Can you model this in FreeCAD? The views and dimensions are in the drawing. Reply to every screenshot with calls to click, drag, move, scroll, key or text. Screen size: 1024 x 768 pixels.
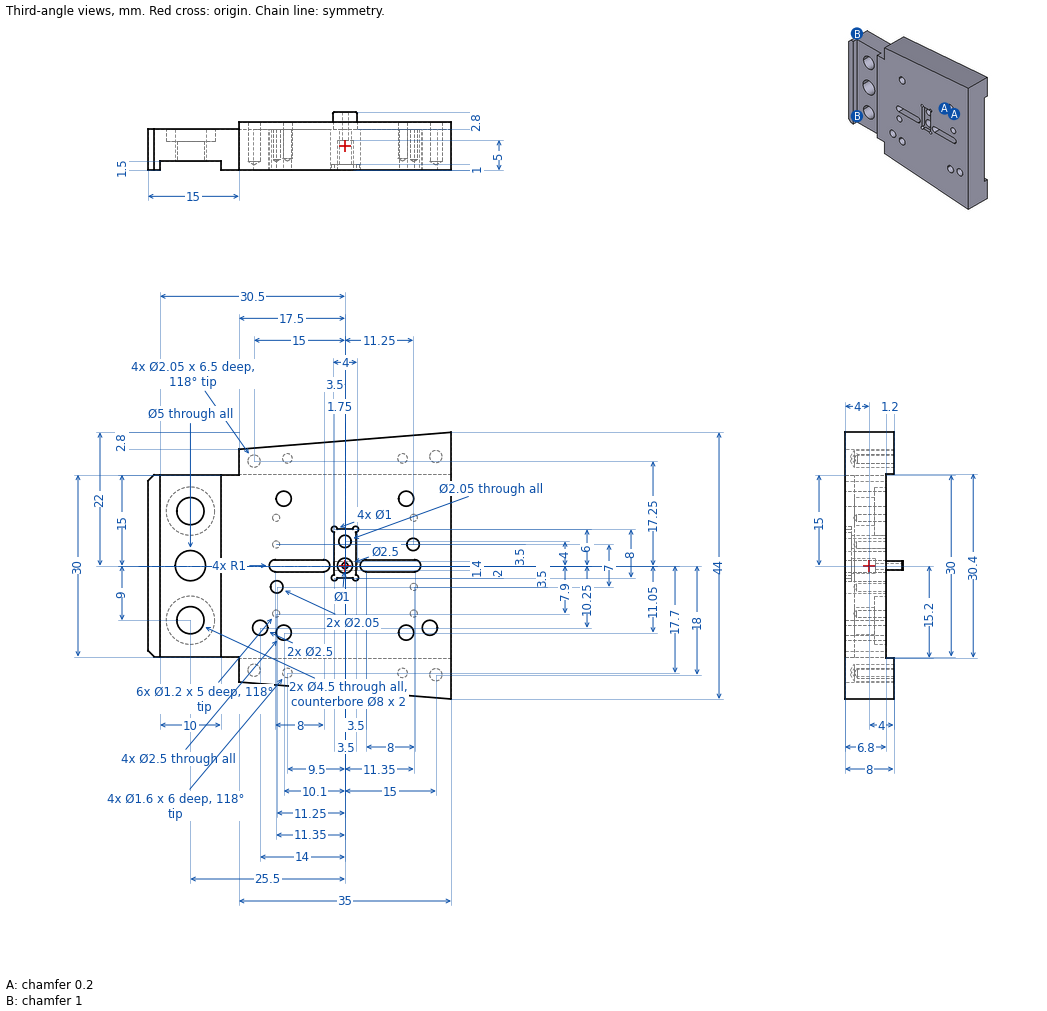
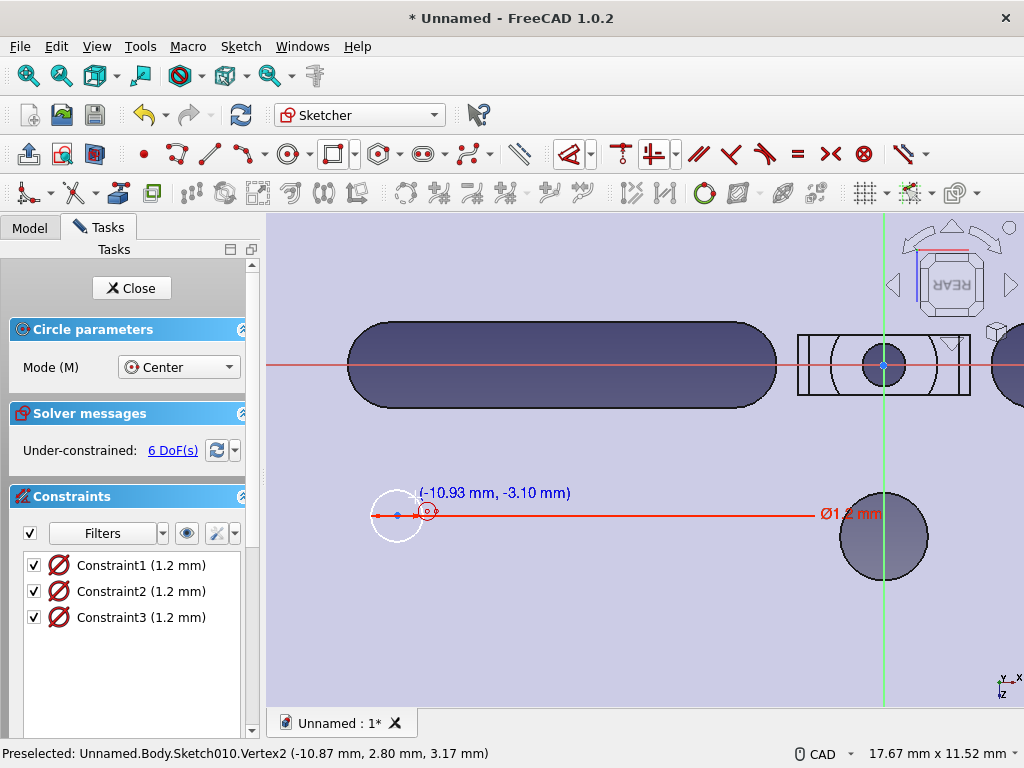
scroll(398, 515, down, 5)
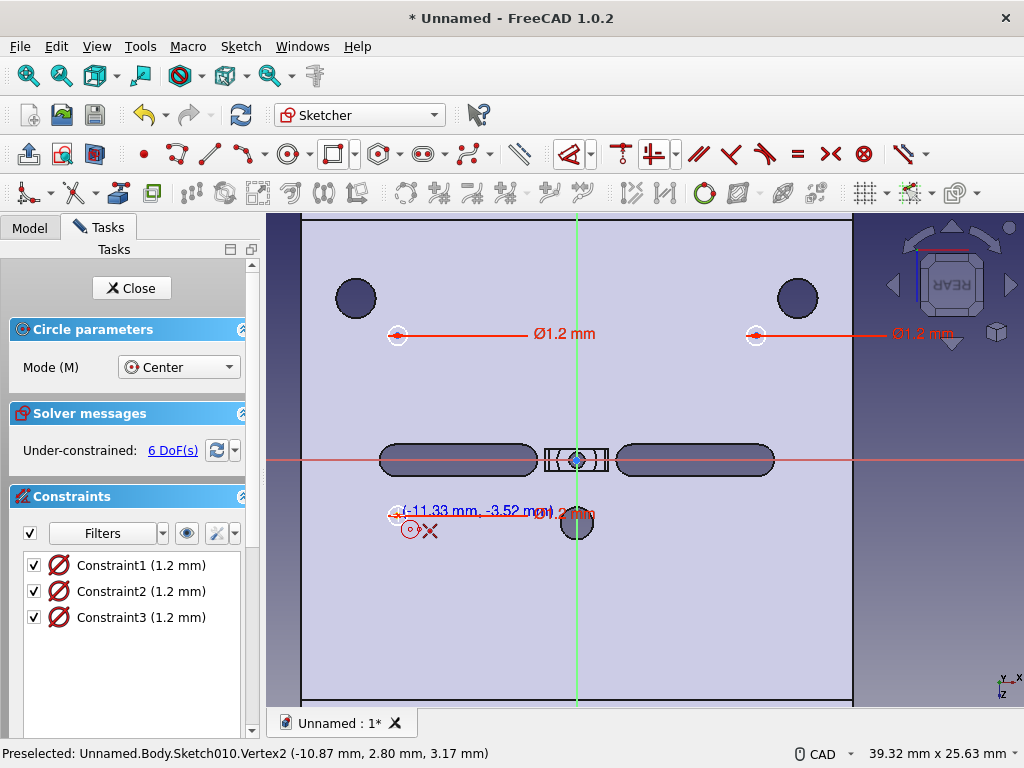
scroll(756, 405, up, 5)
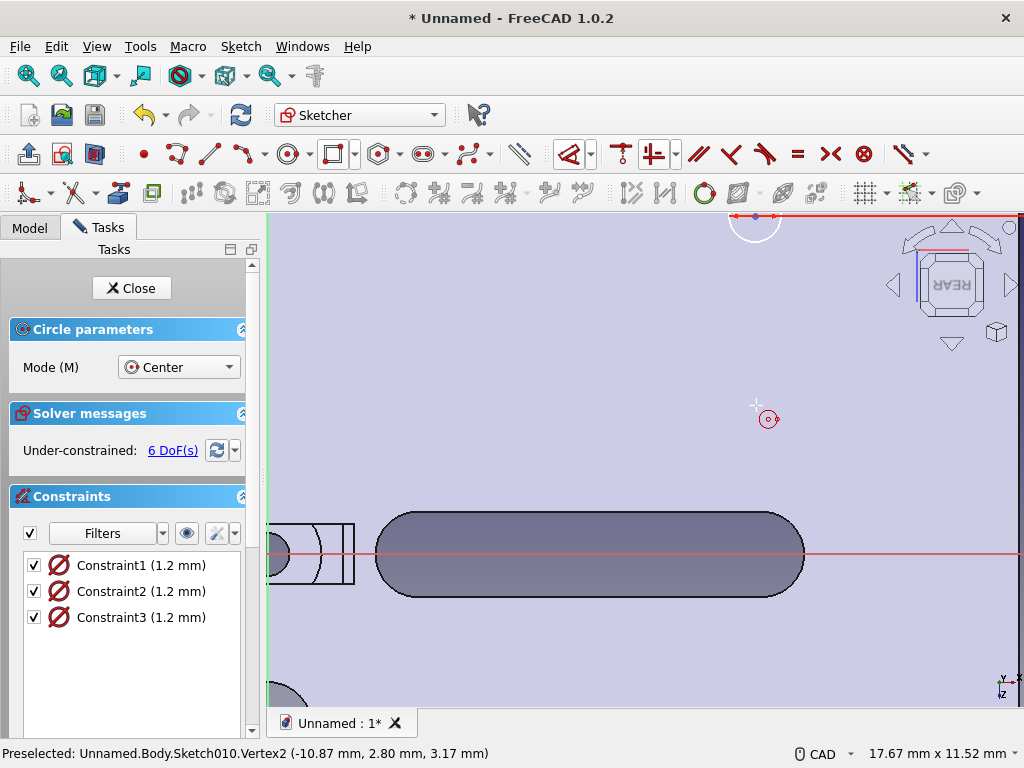
click(755, 404)
move(773, 386)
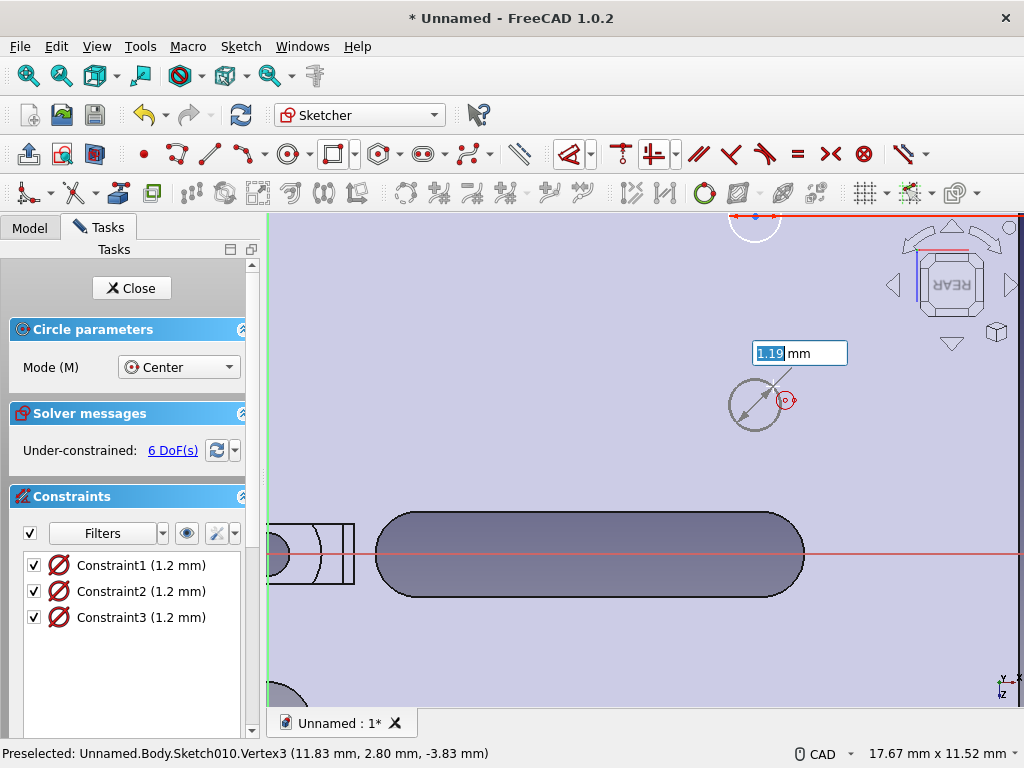
text(1.2)
key(Return)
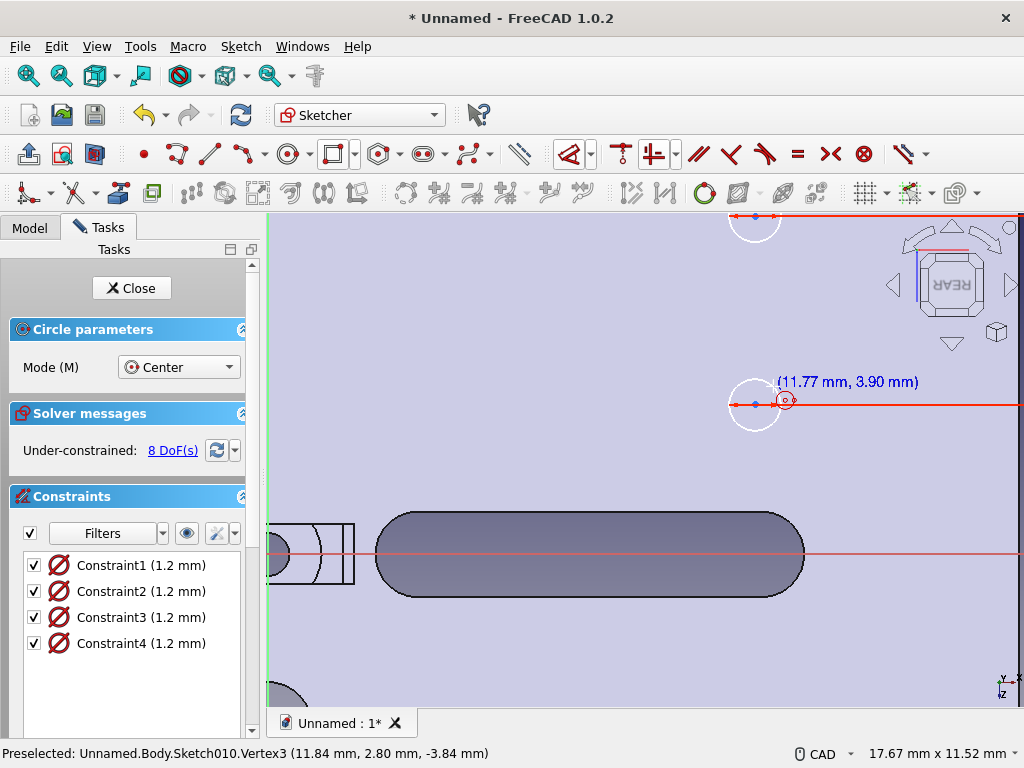
scroll(756, 405, down, 5)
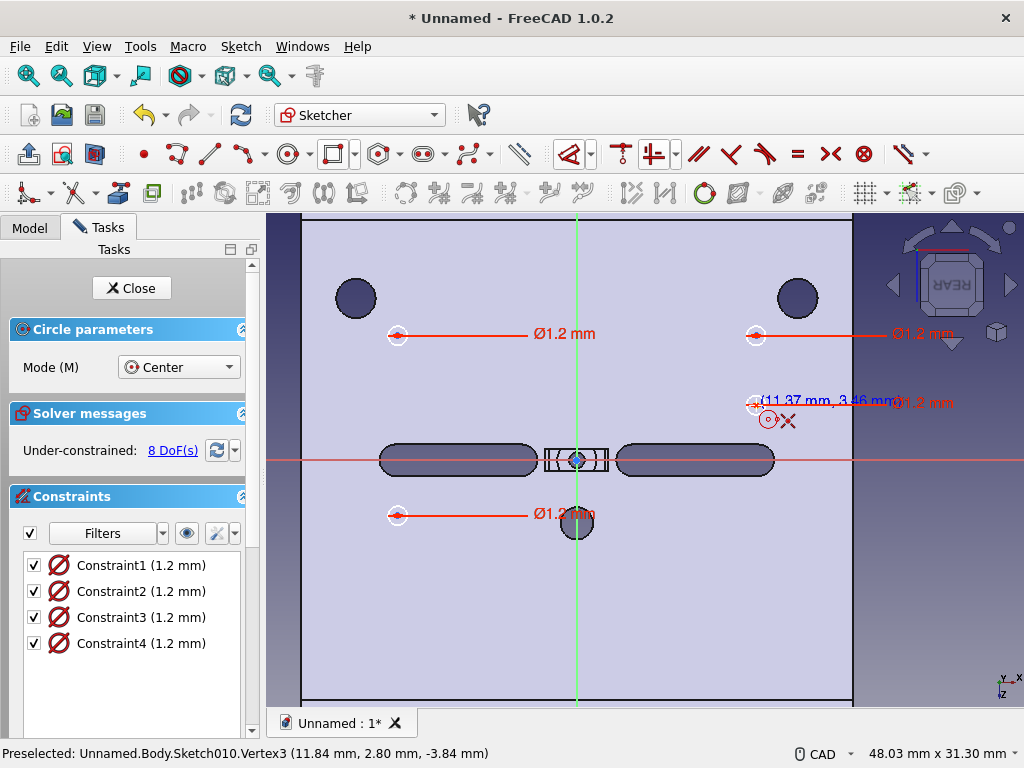
scroll(756, 585, up, 5)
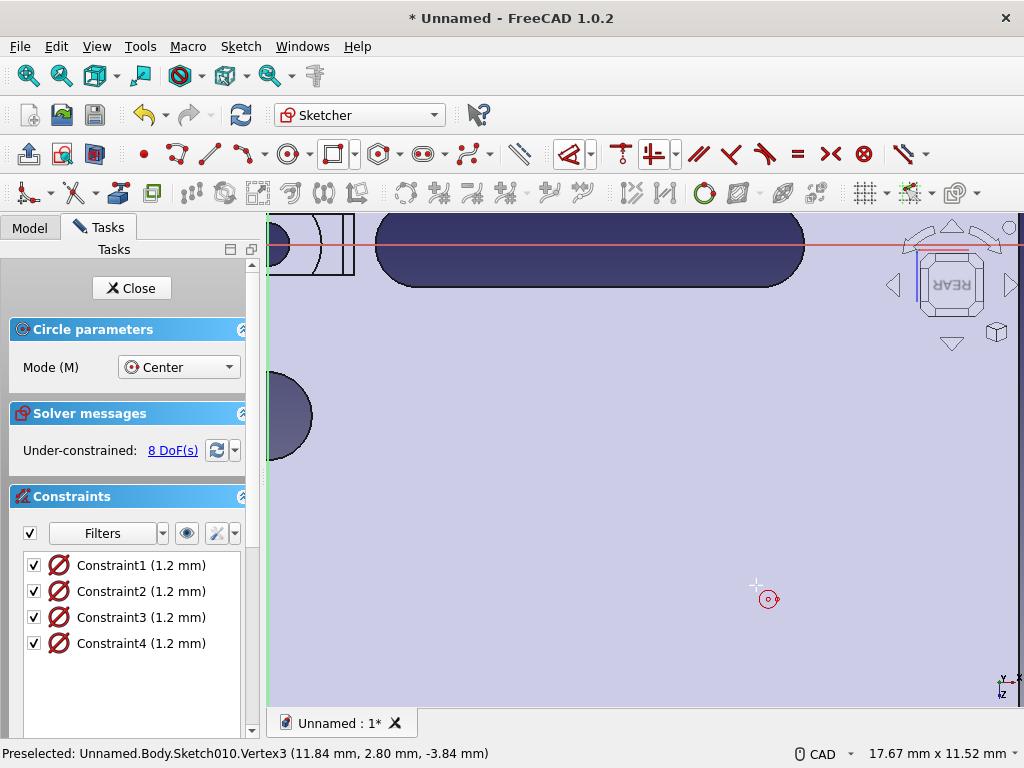
click(755, 583)
move(773, 565)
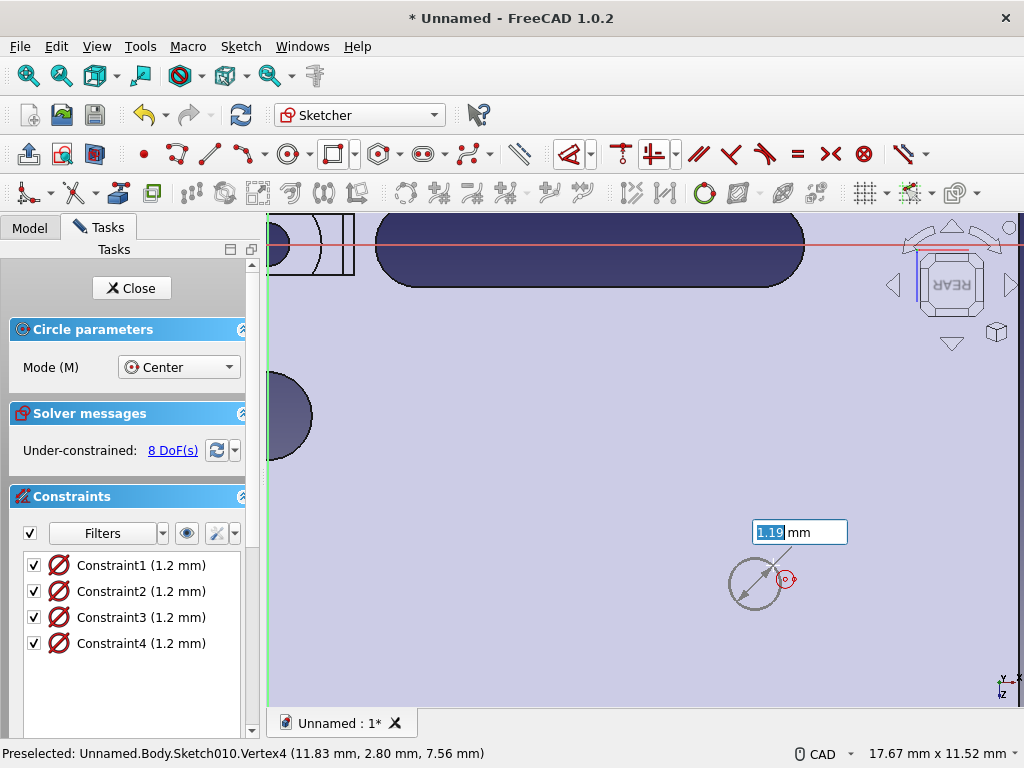
text(1.2)
key(Return)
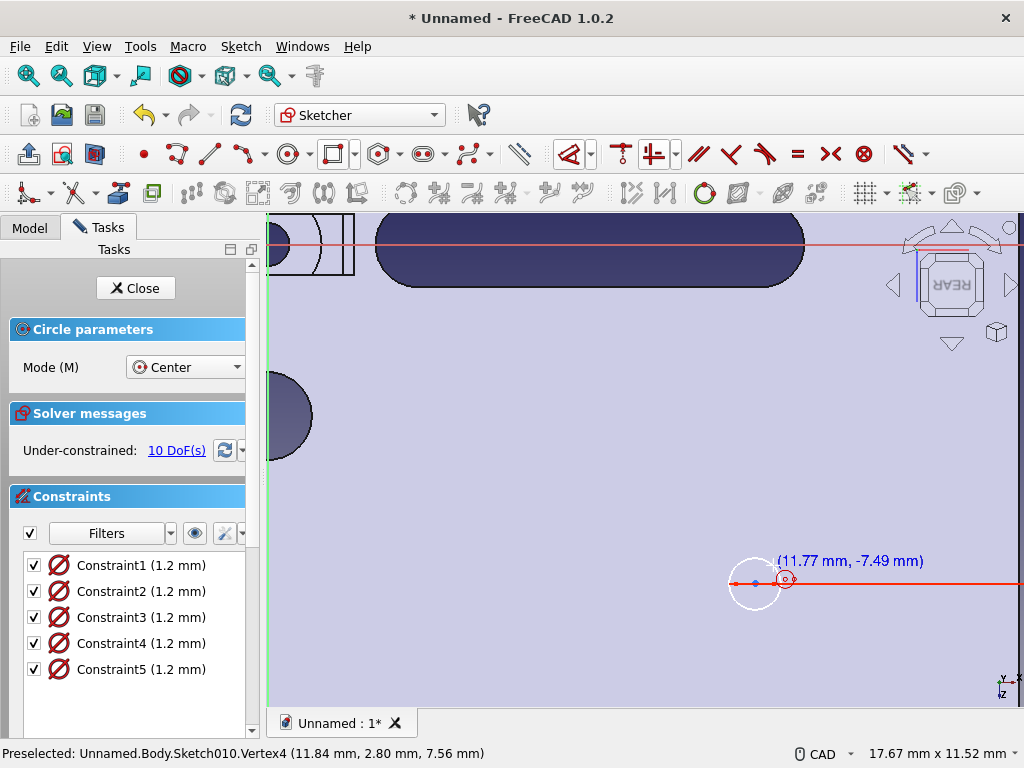
scroll(756, 585, down, 5)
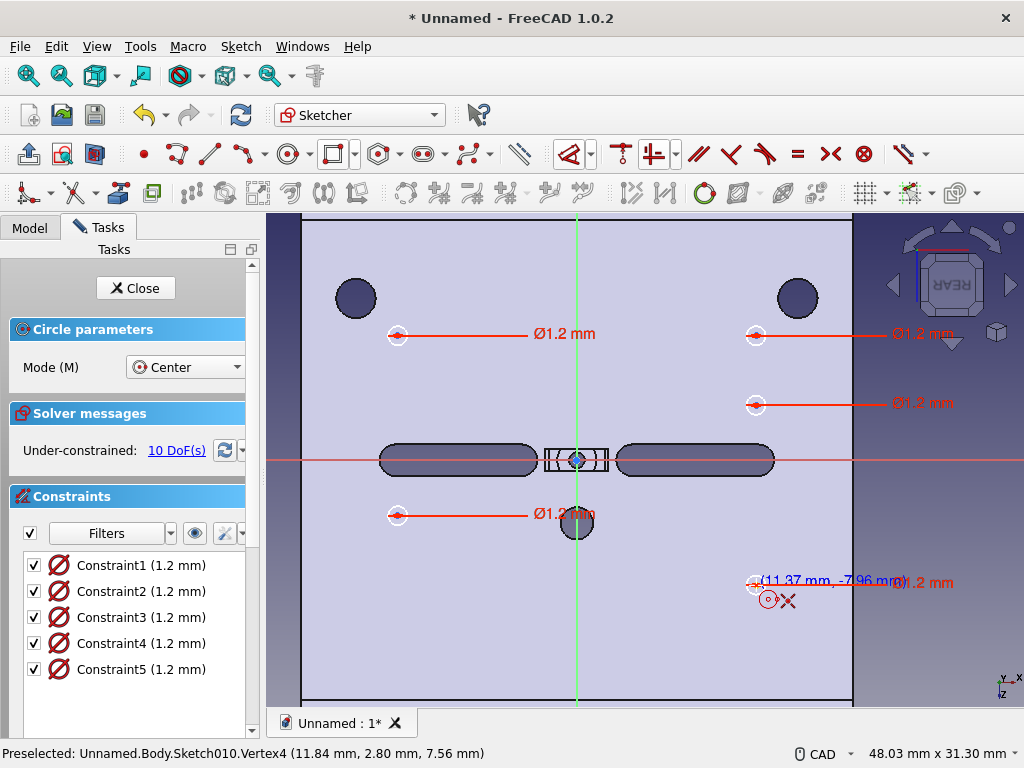
scroll(398, 585, up, 5)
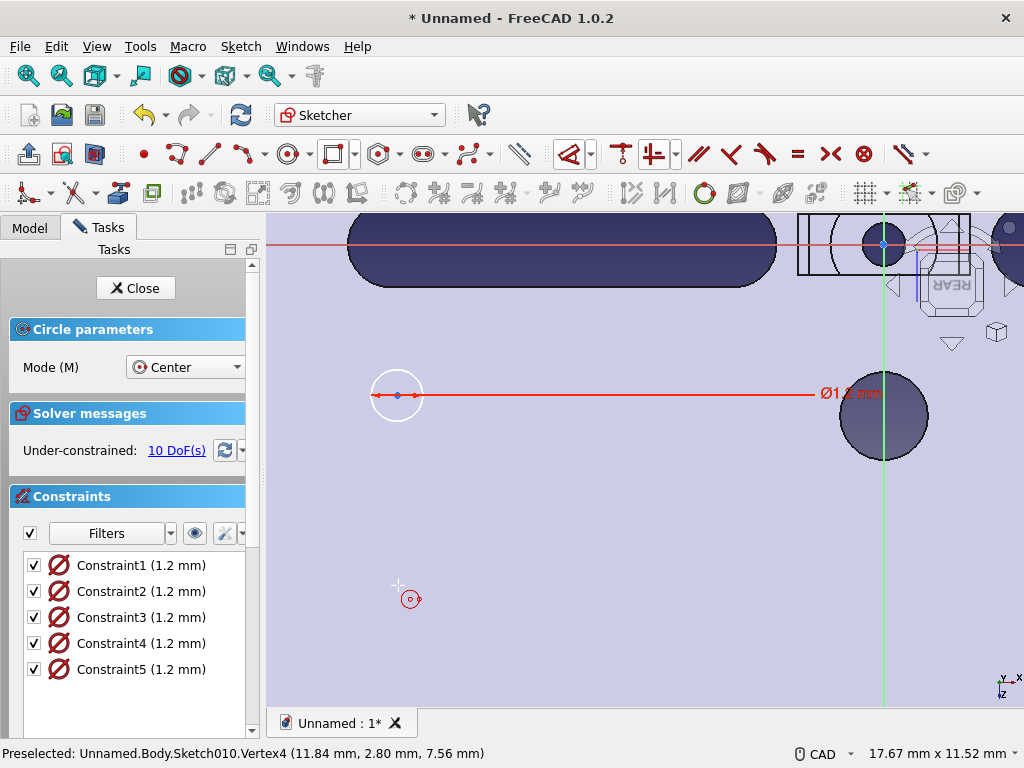
click(397, 583)
move(415, 565)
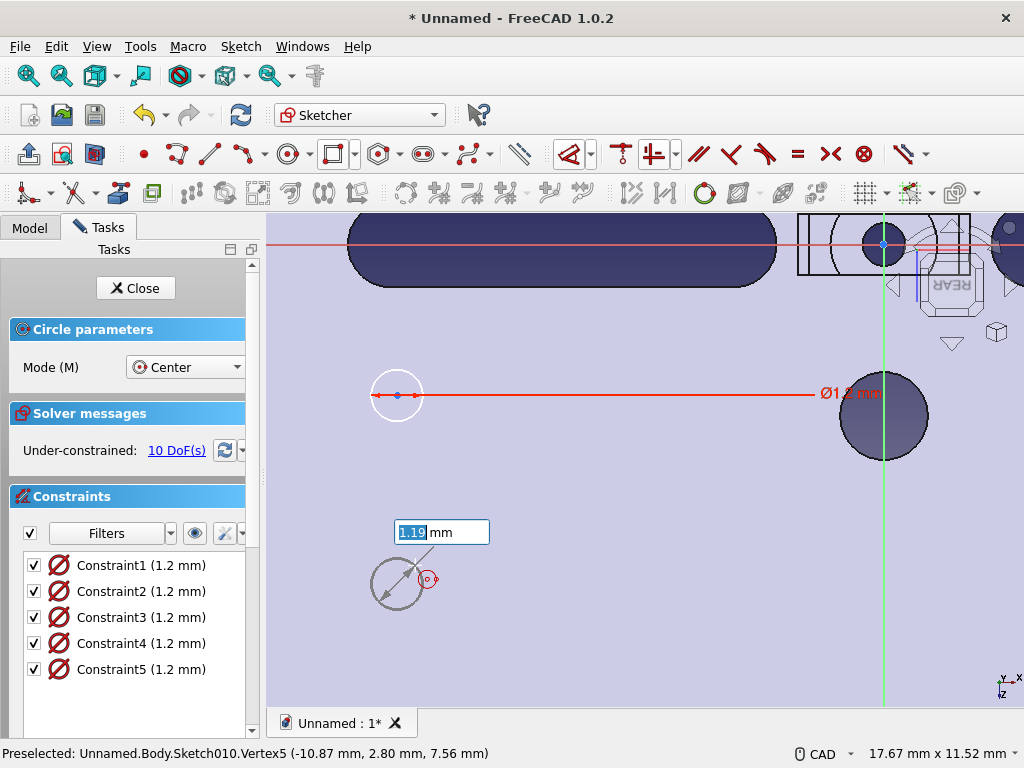
text(1.2)
key(Return)
key(Escape)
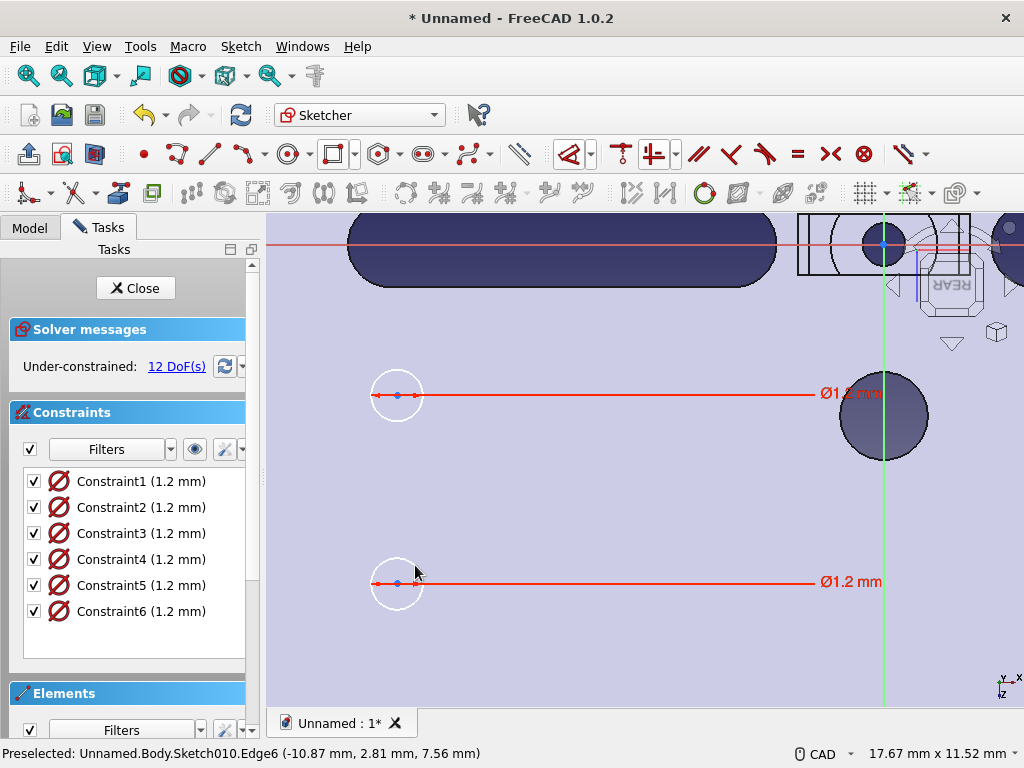
scroll(398, 585, down, 5)